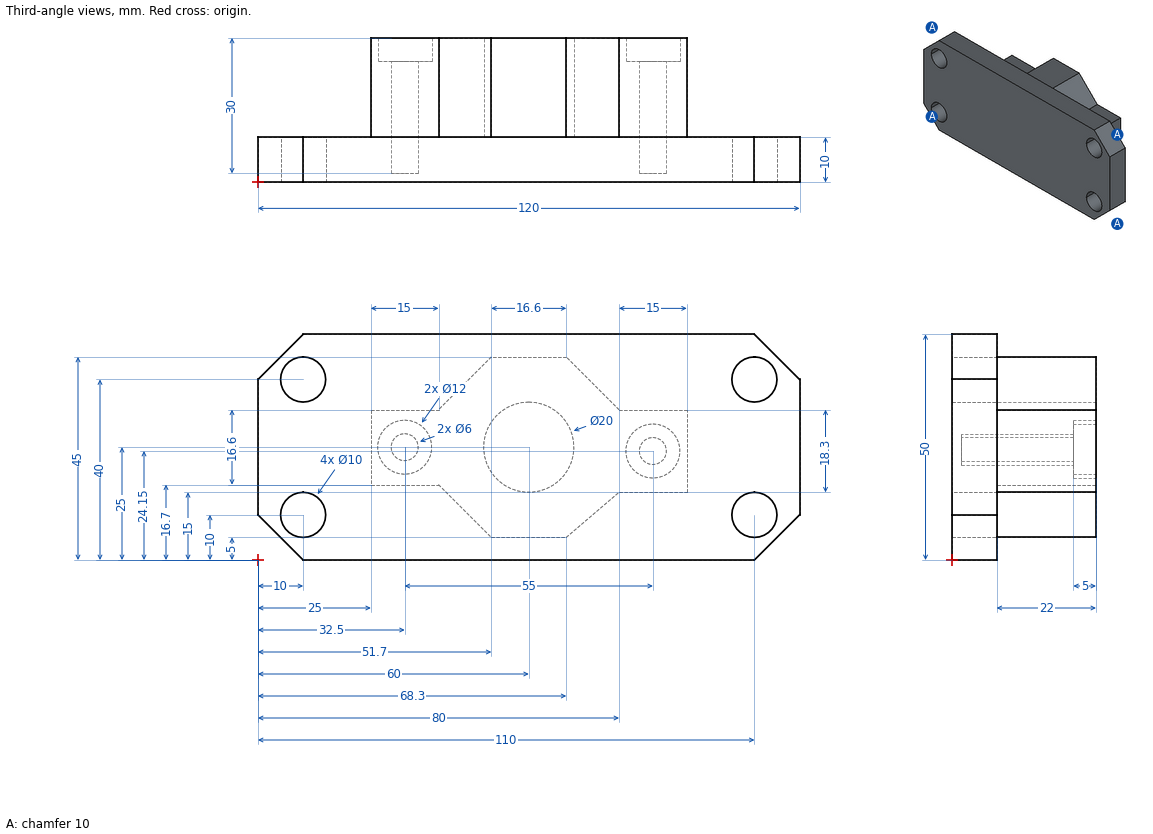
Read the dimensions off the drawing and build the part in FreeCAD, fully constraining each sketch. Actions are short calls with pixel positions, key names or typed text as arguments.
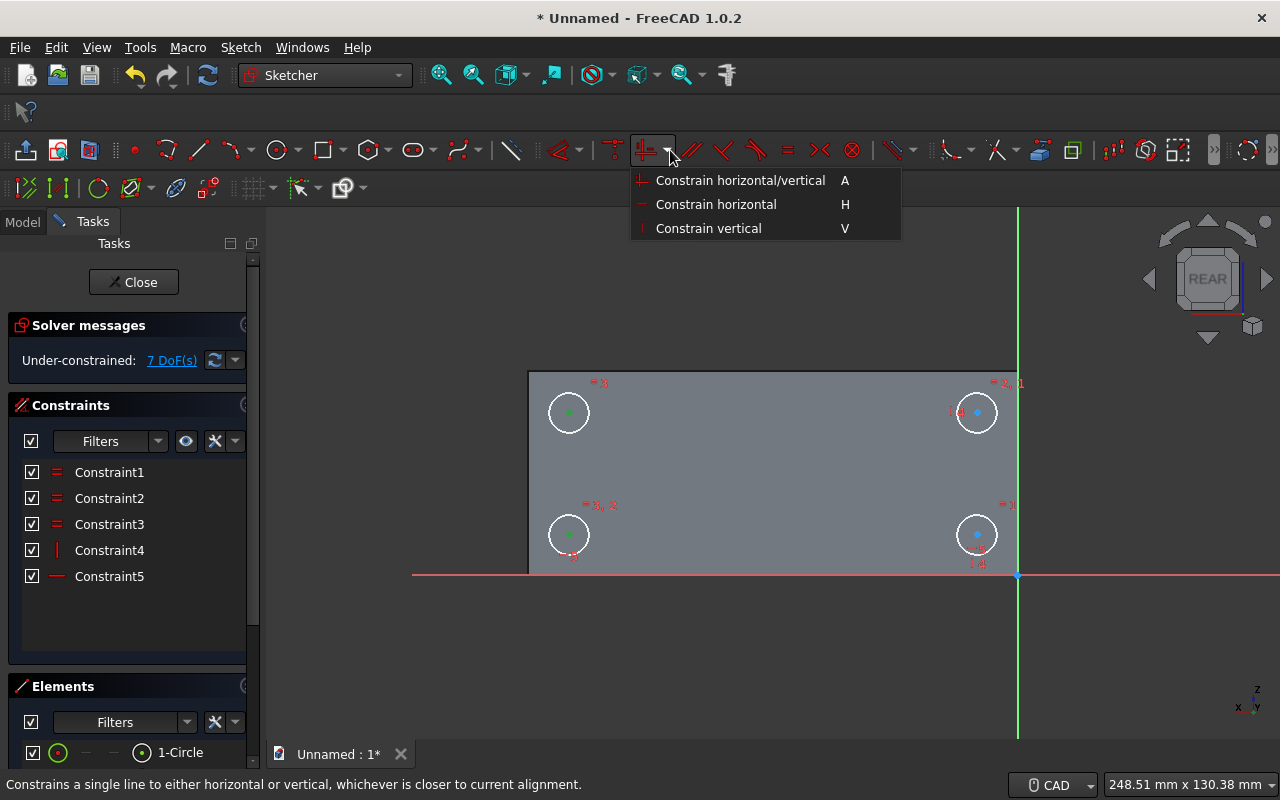
click(766, 228)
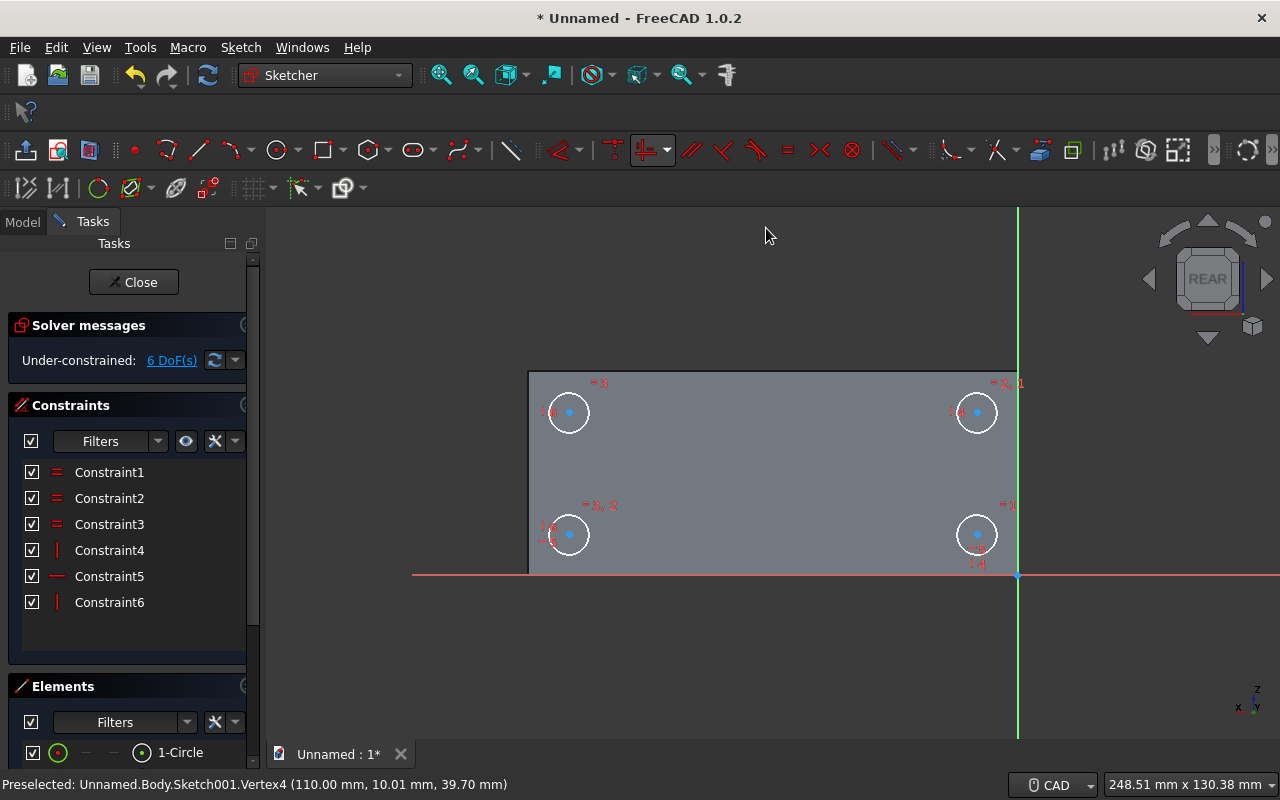
click(977, 413)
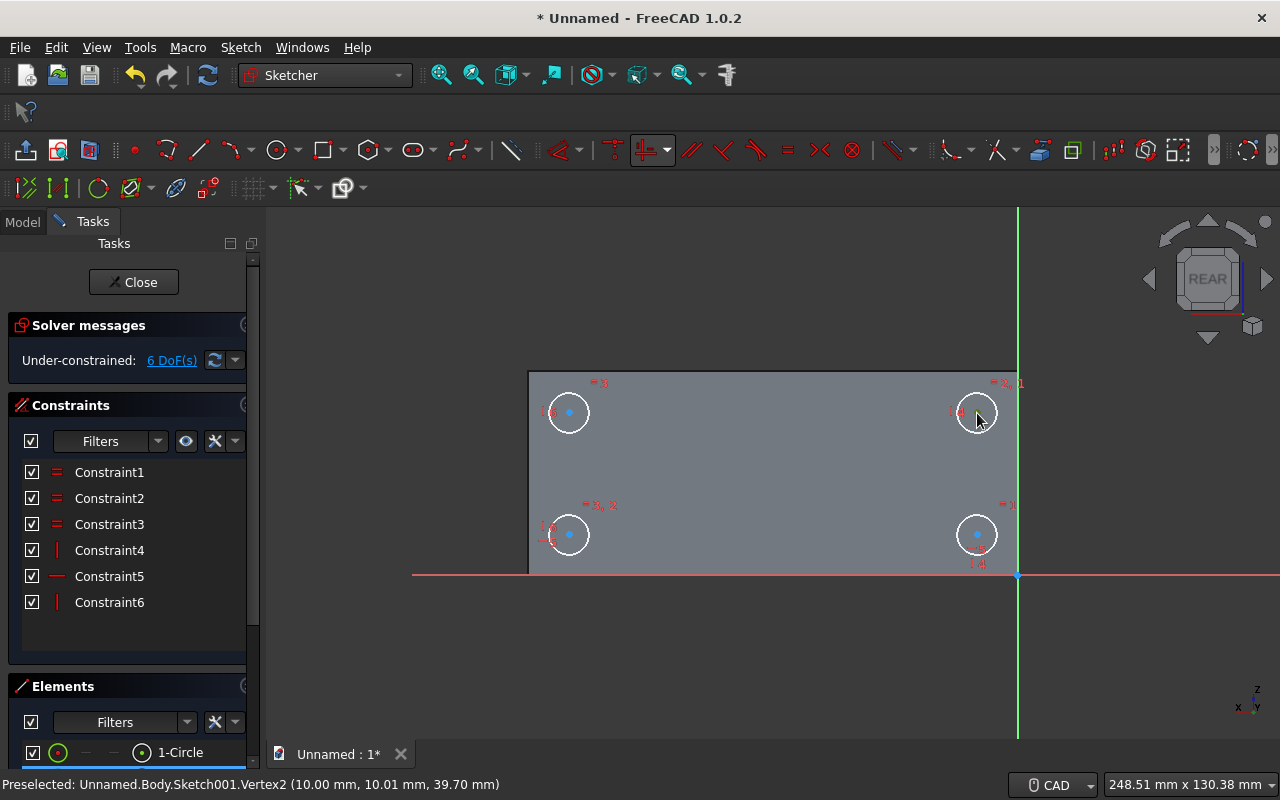
click(569, 413)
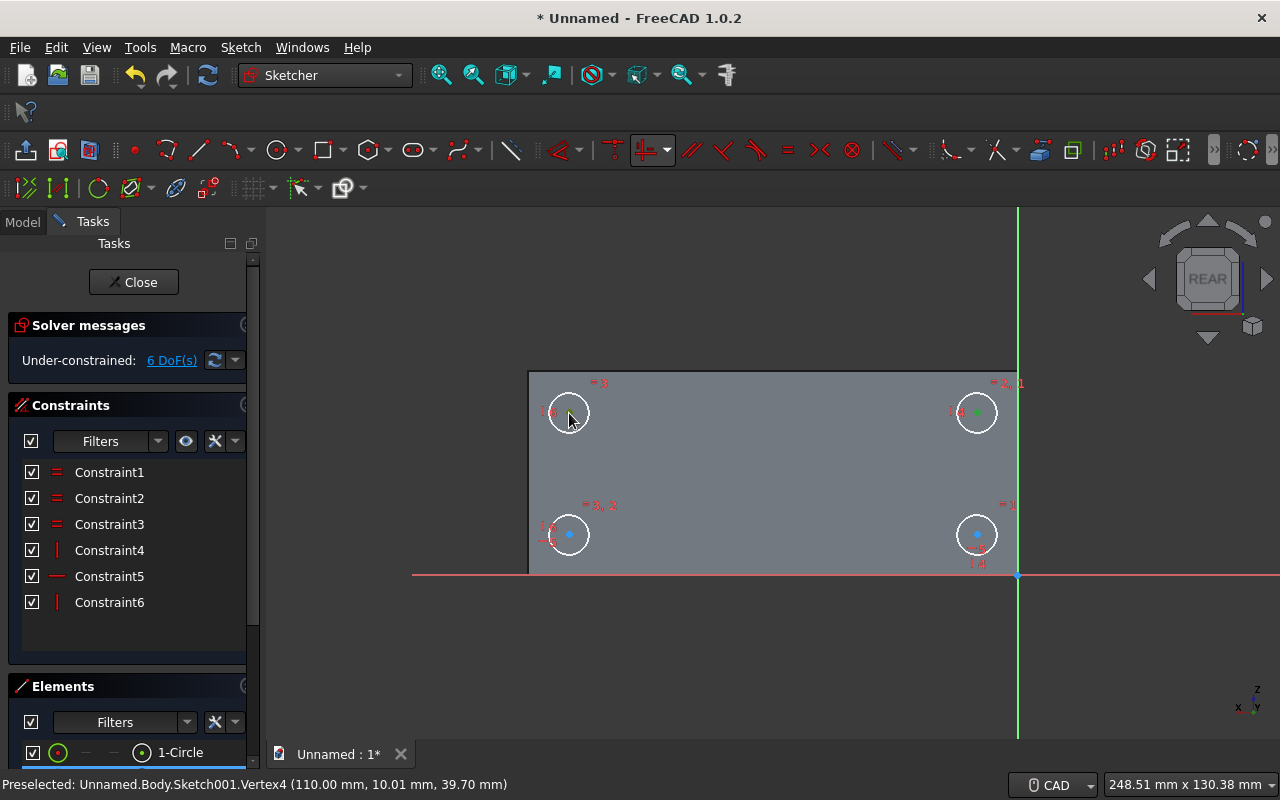
click(670, 150)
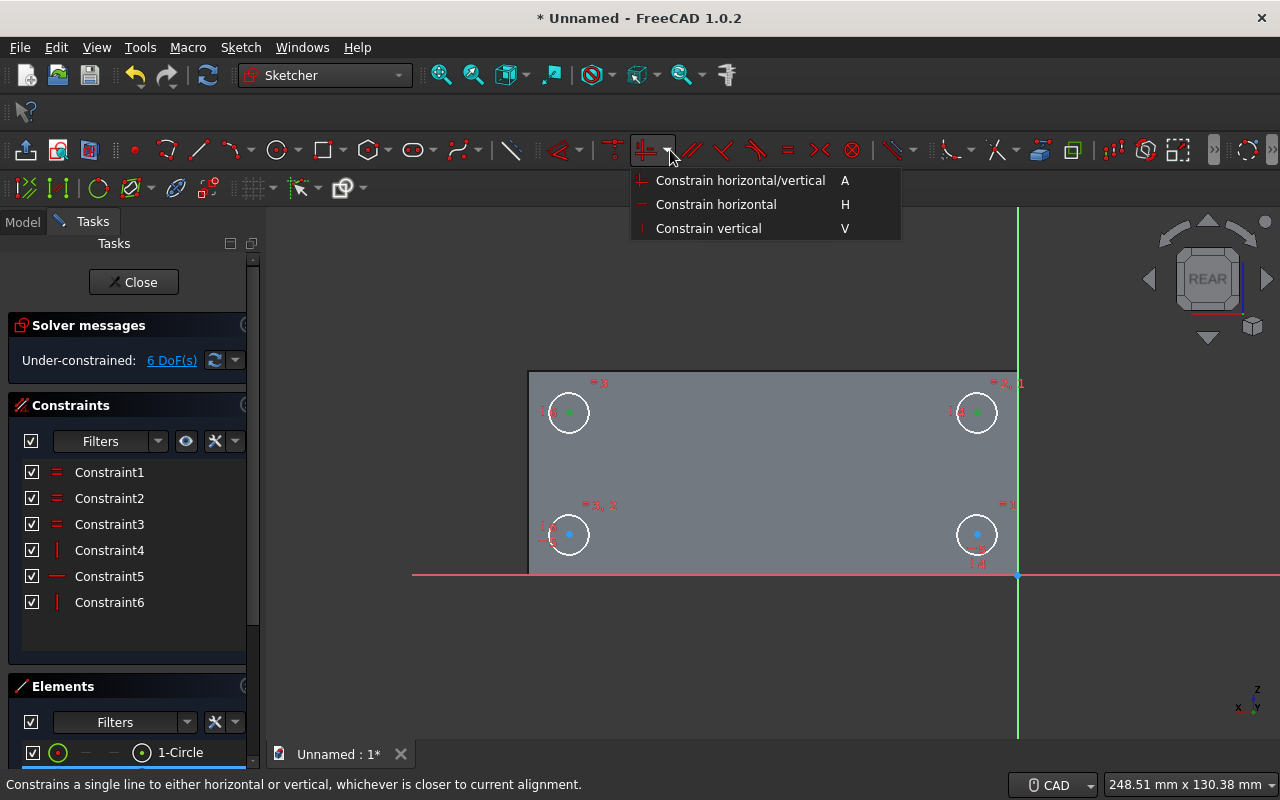
click(766, 204)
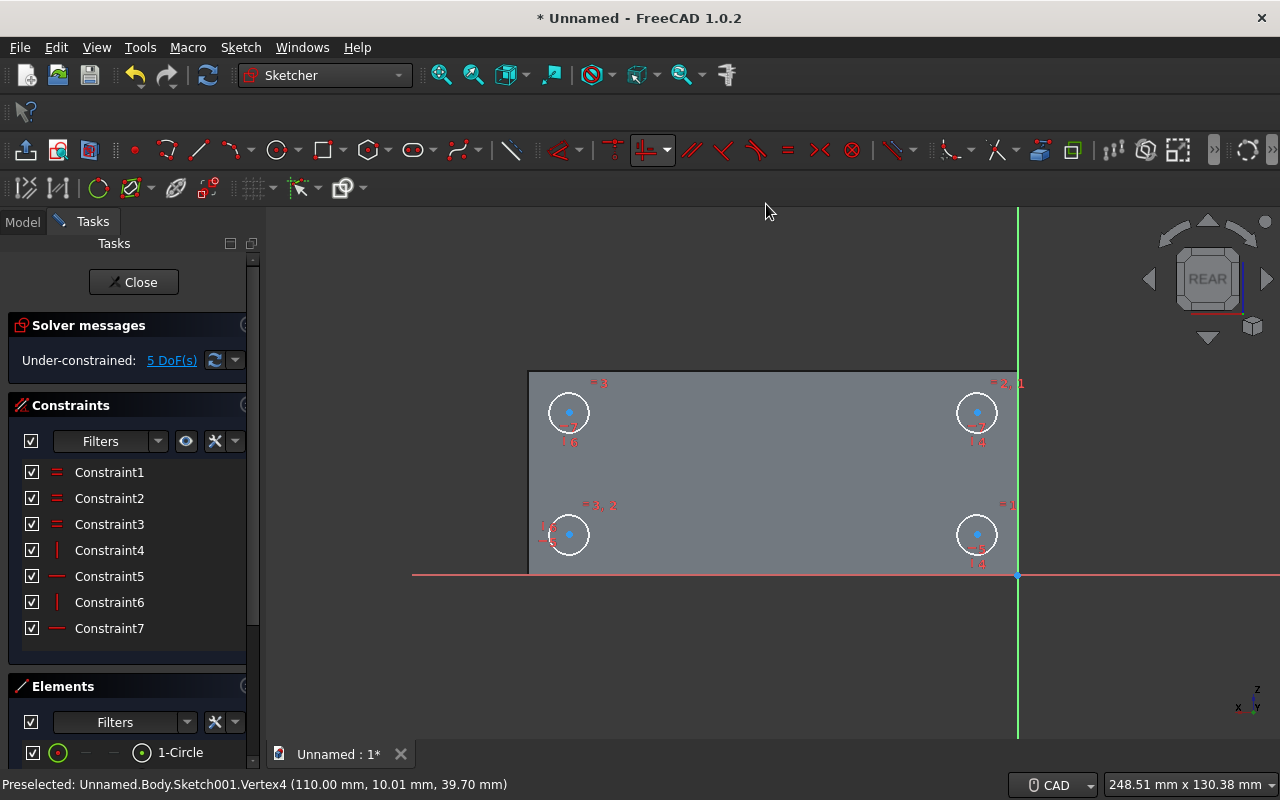
click(558, 150)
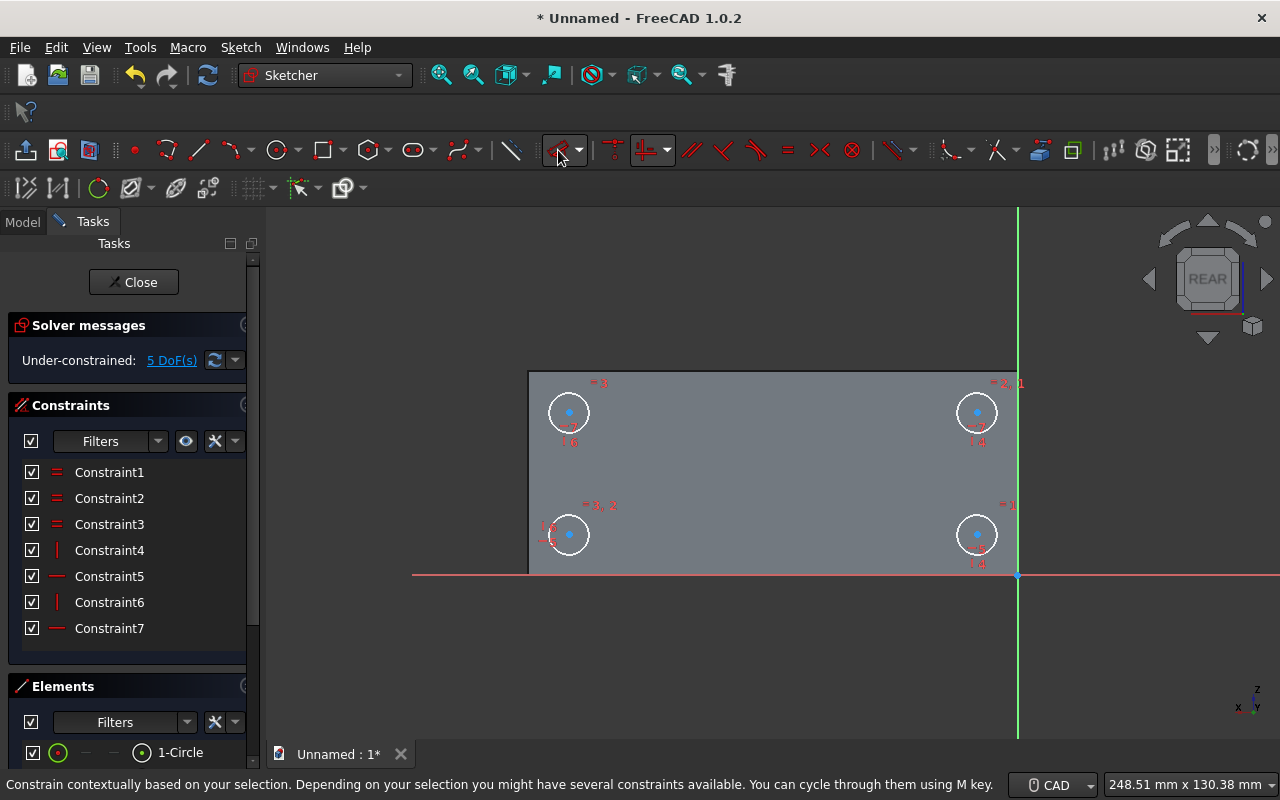
click(991, 521)
click(992, 485)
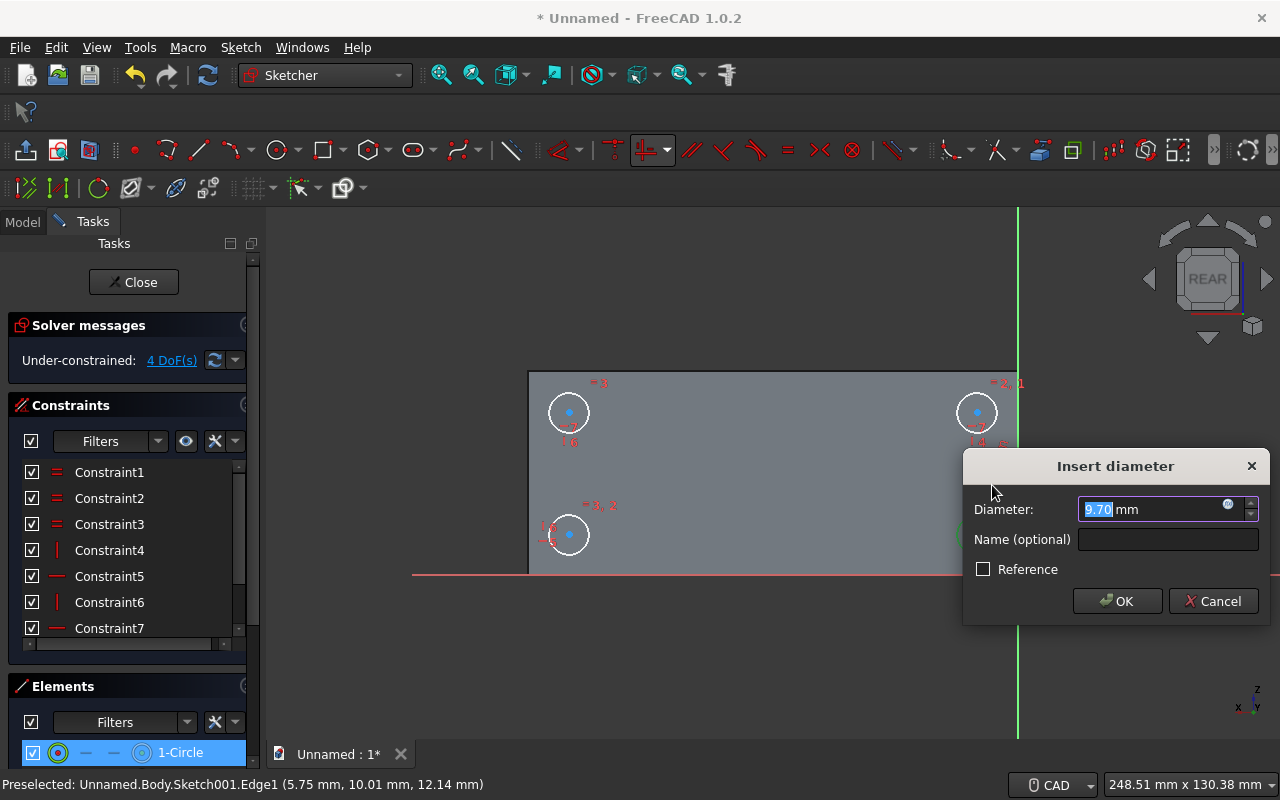
text(10)
key(Return)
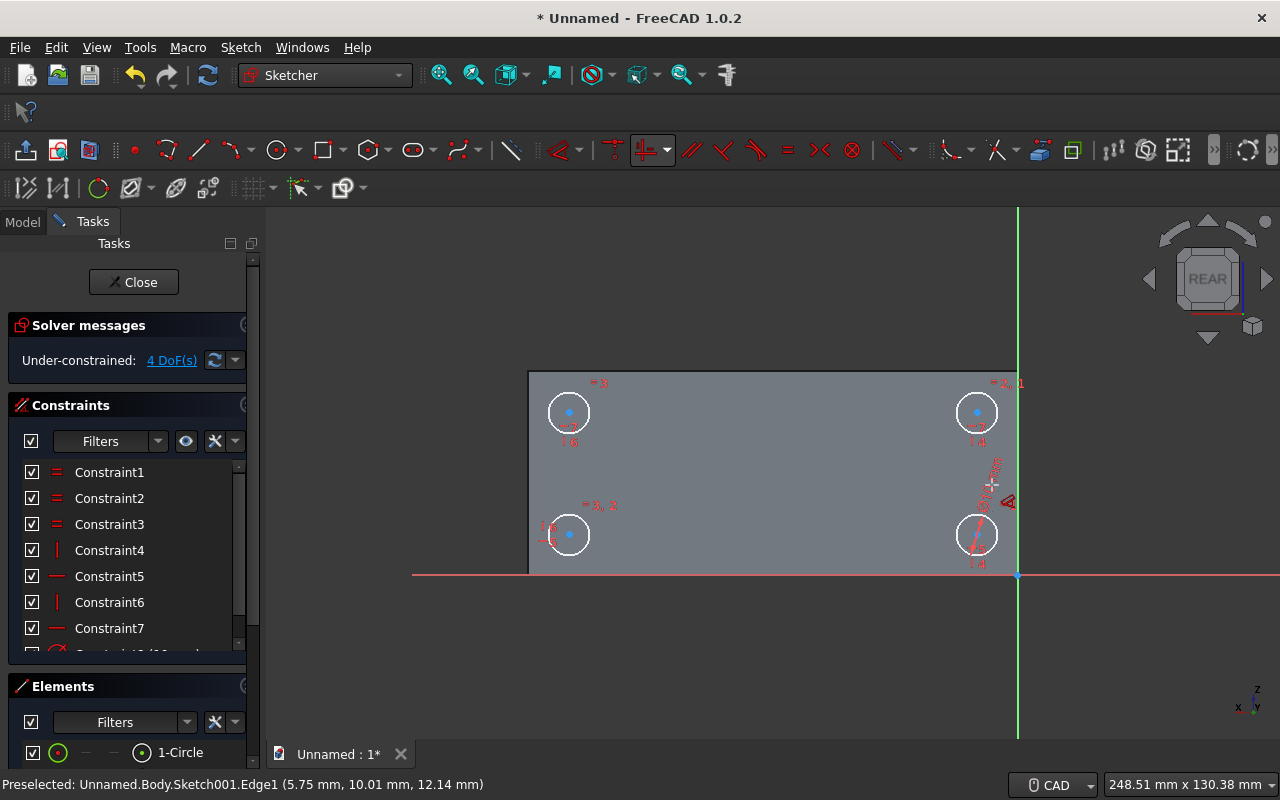
click(977, 535)
click(997, 609)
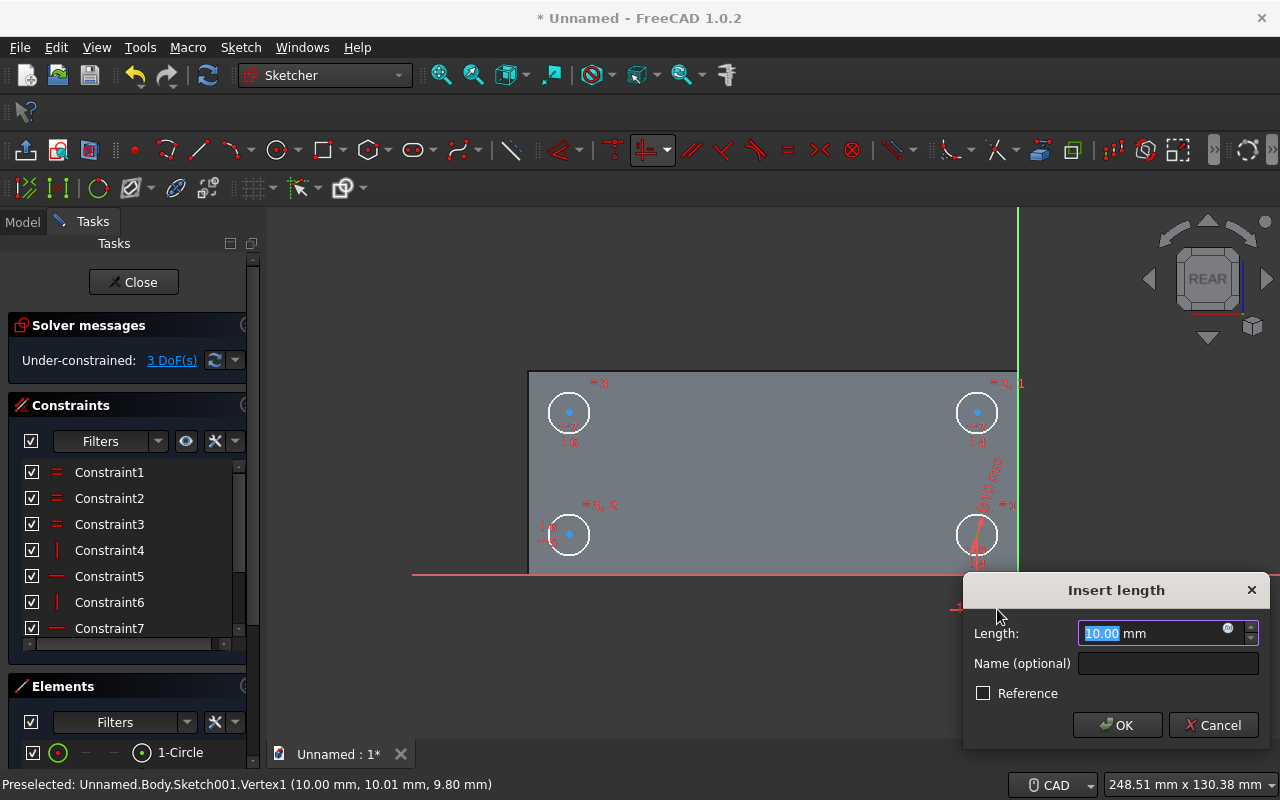
text(10)
key(Return)